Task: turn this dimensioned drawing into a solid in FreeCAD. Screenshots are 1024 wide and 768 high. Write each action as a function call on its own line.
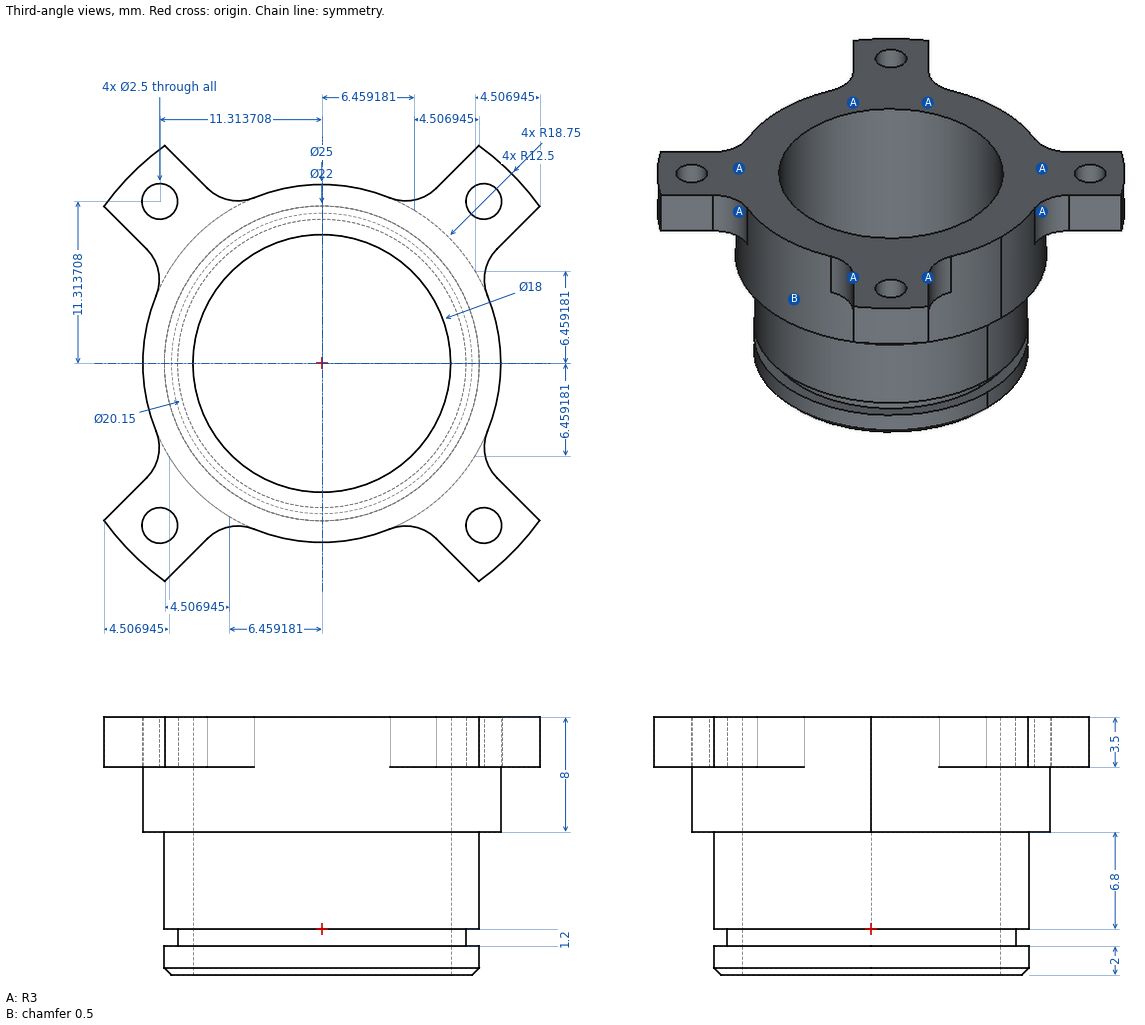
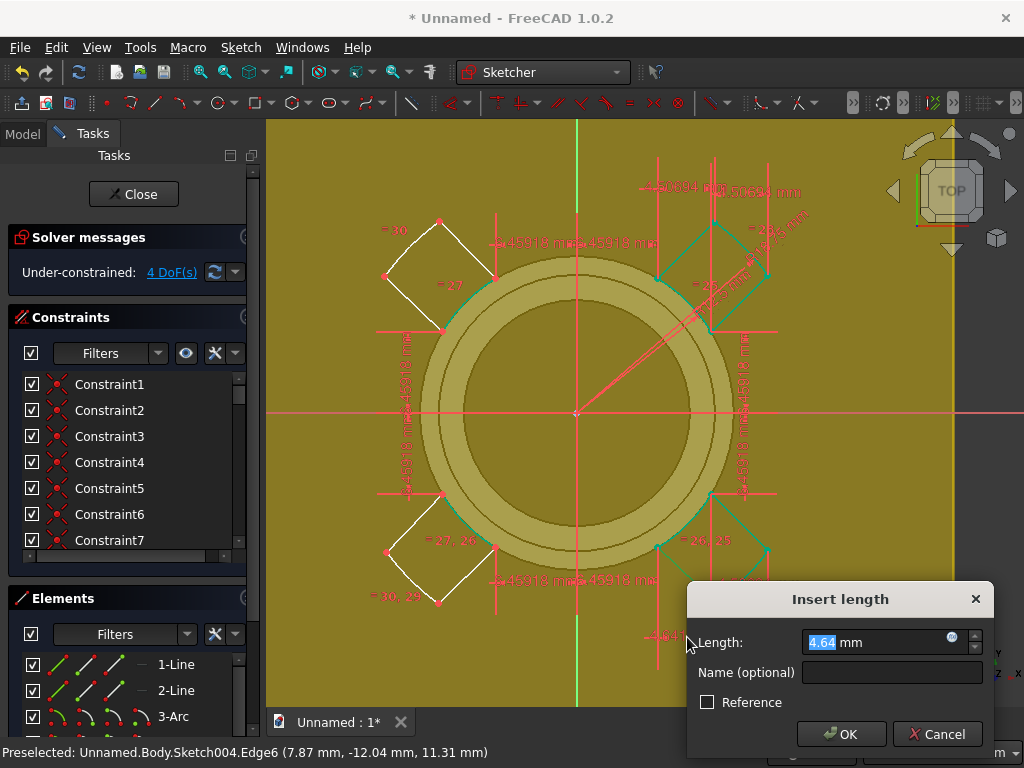
text(4.506945)
key(Return)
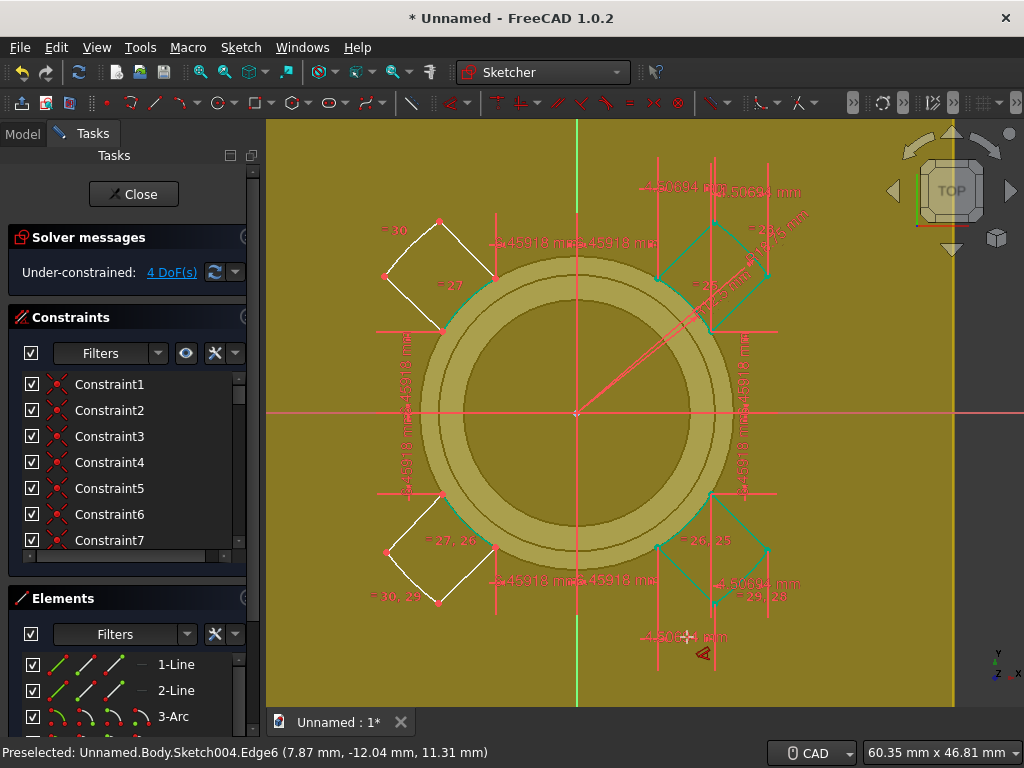
click(456, 587)
click(467, 638)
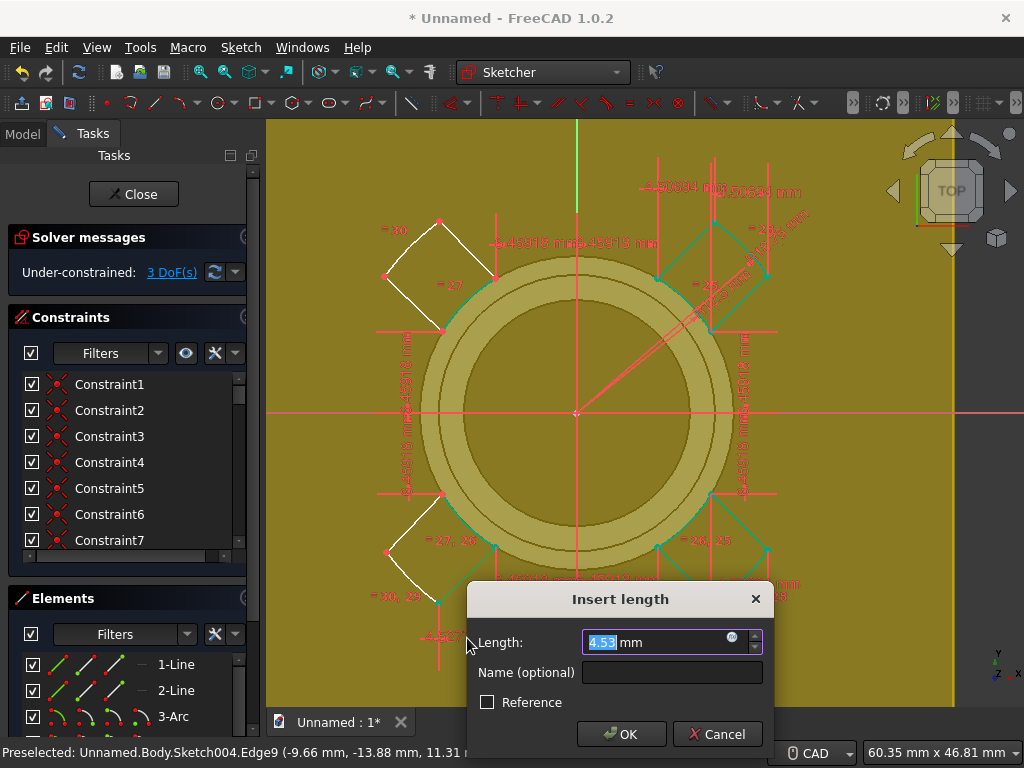
text(4.506945)
key(Return)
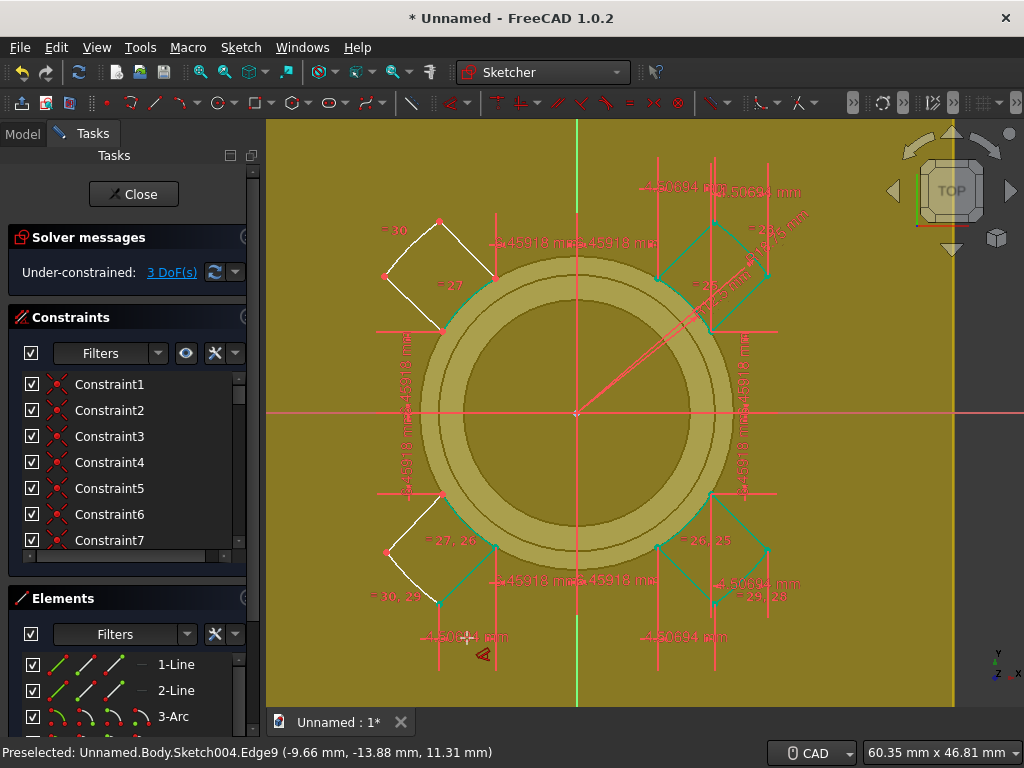
click(426, 512)
click(395, 586)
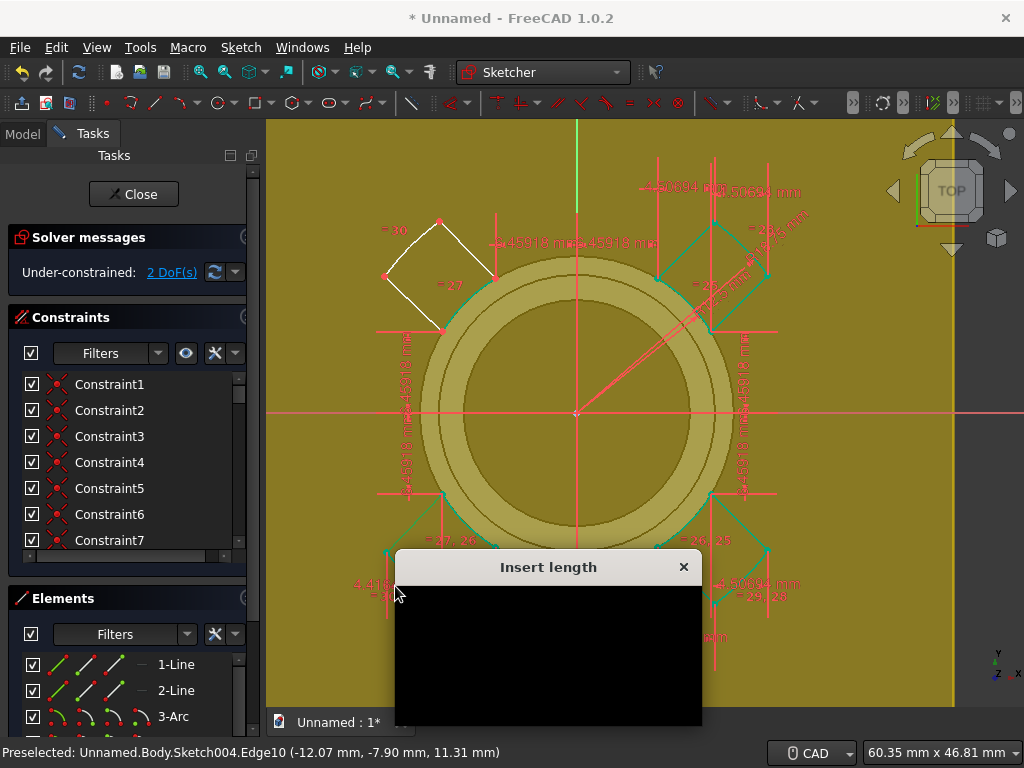
text(4.506945)
key(Return)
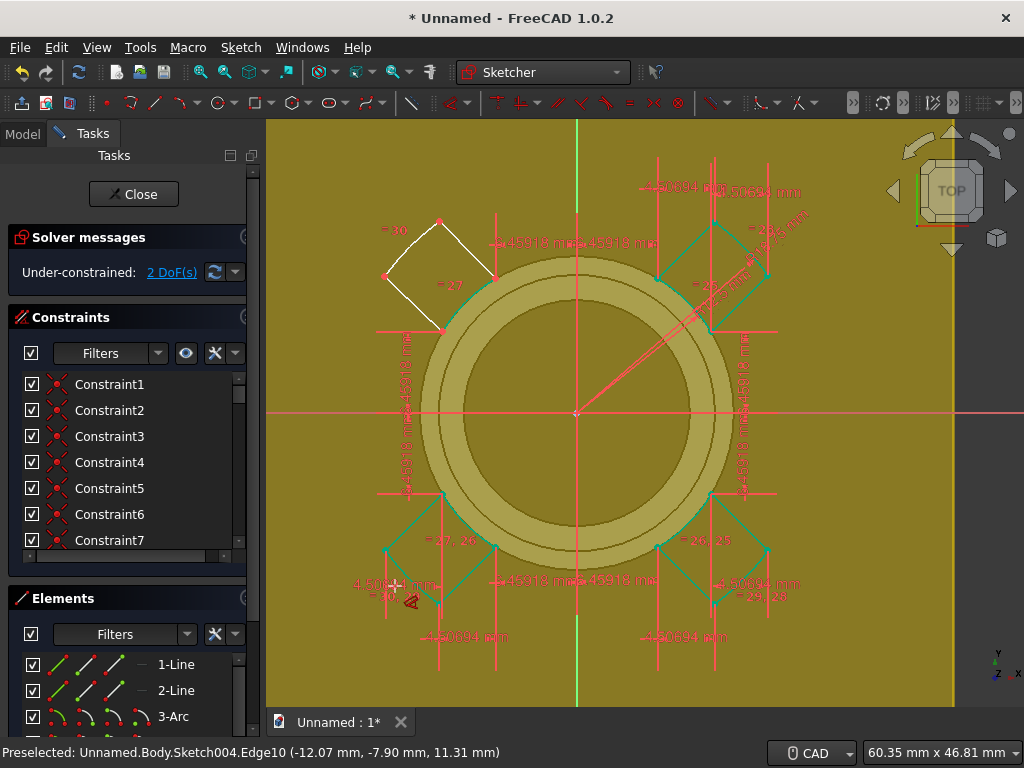
click(402, 293)
click(393, 243)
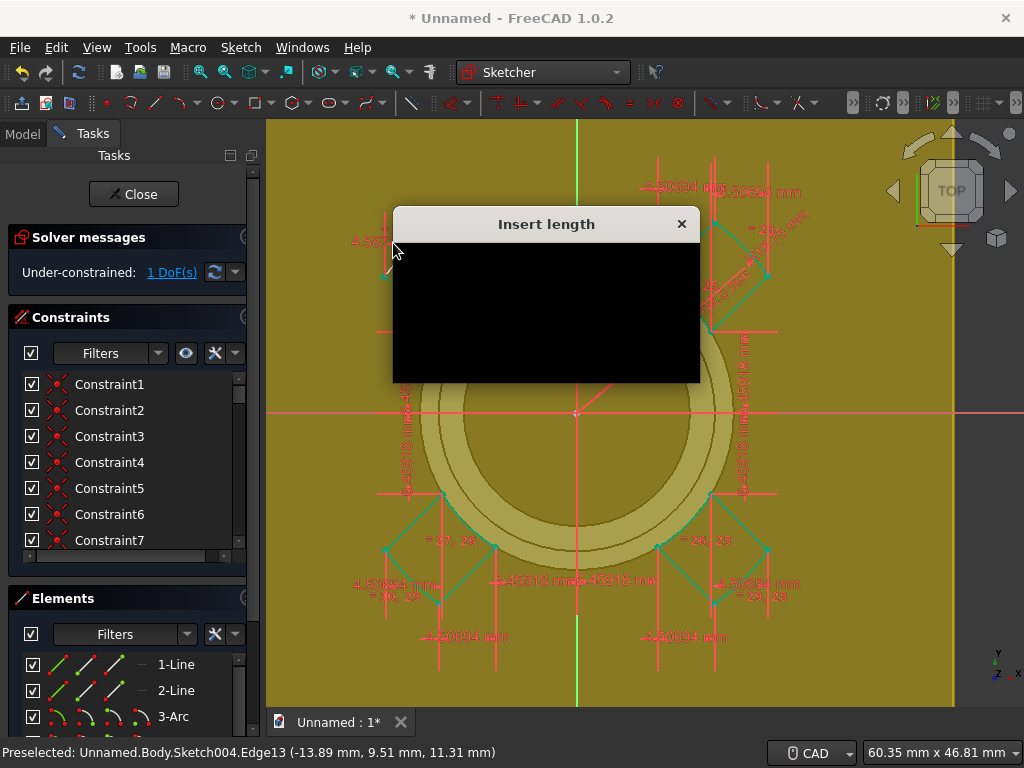
text(4.506945)
key(Return)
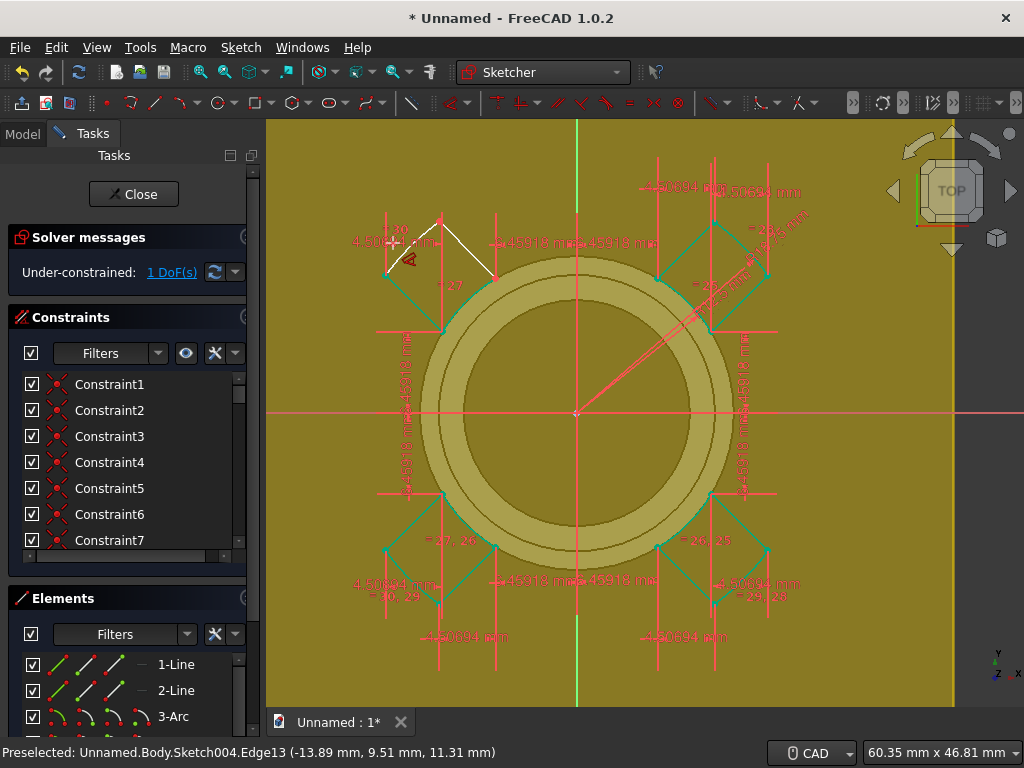
click(479, 262)
click(468, 187)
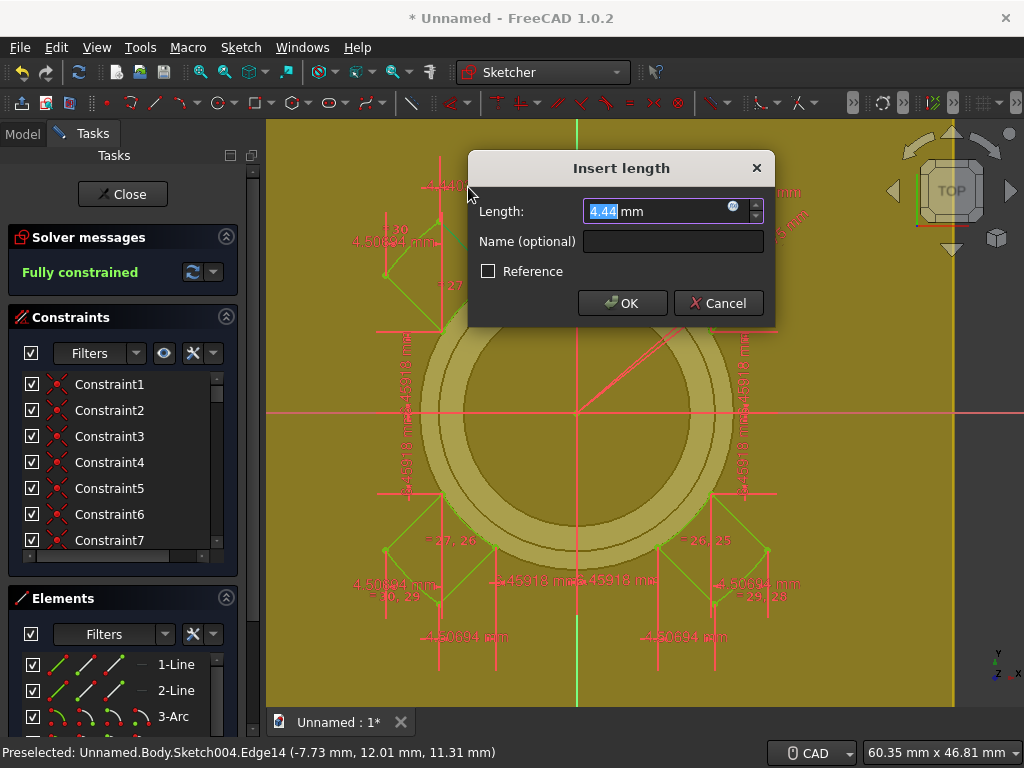
text(4.506945)
key(Return)
key(Escape)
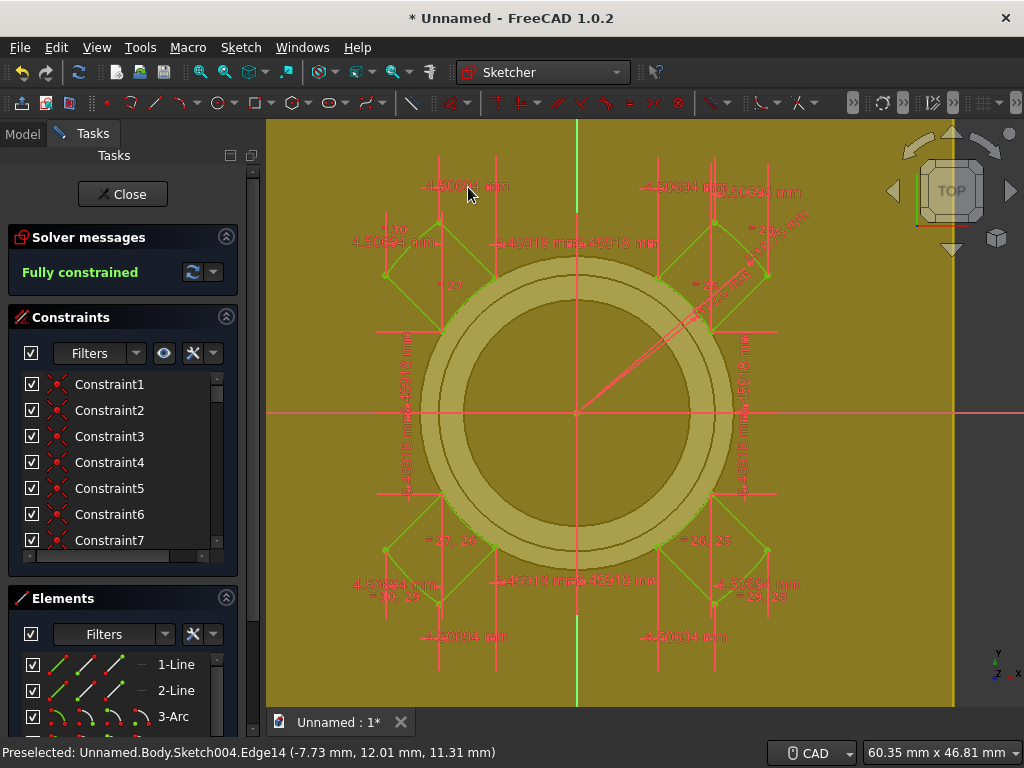
click(123, 194)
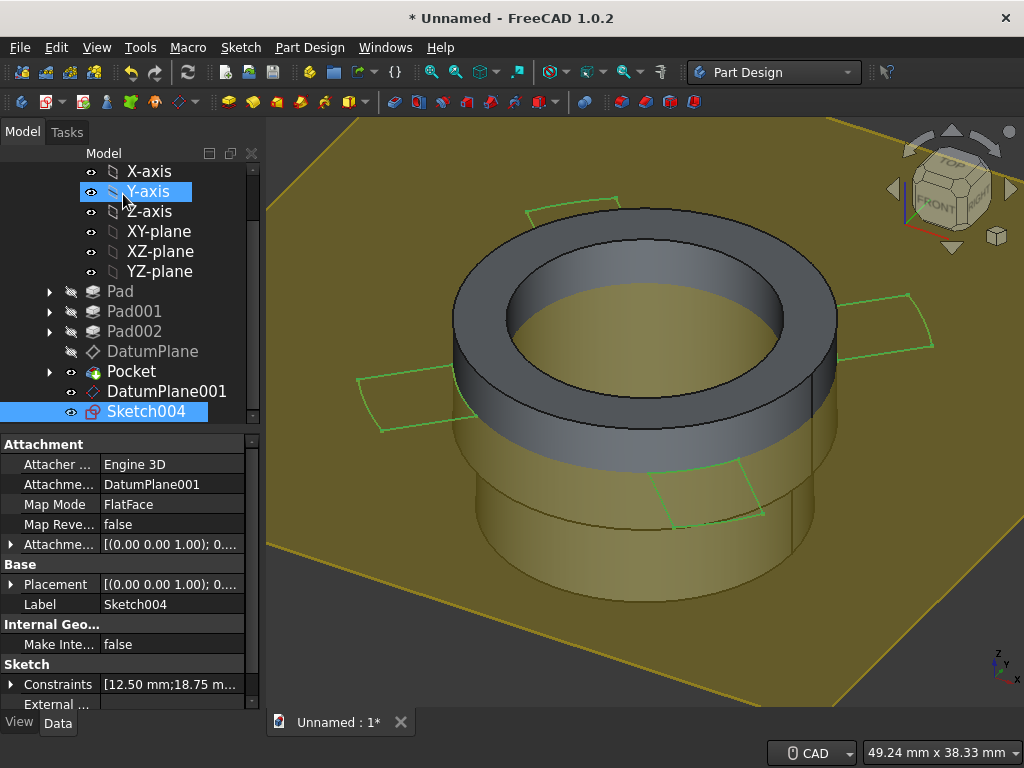
click(230, 102)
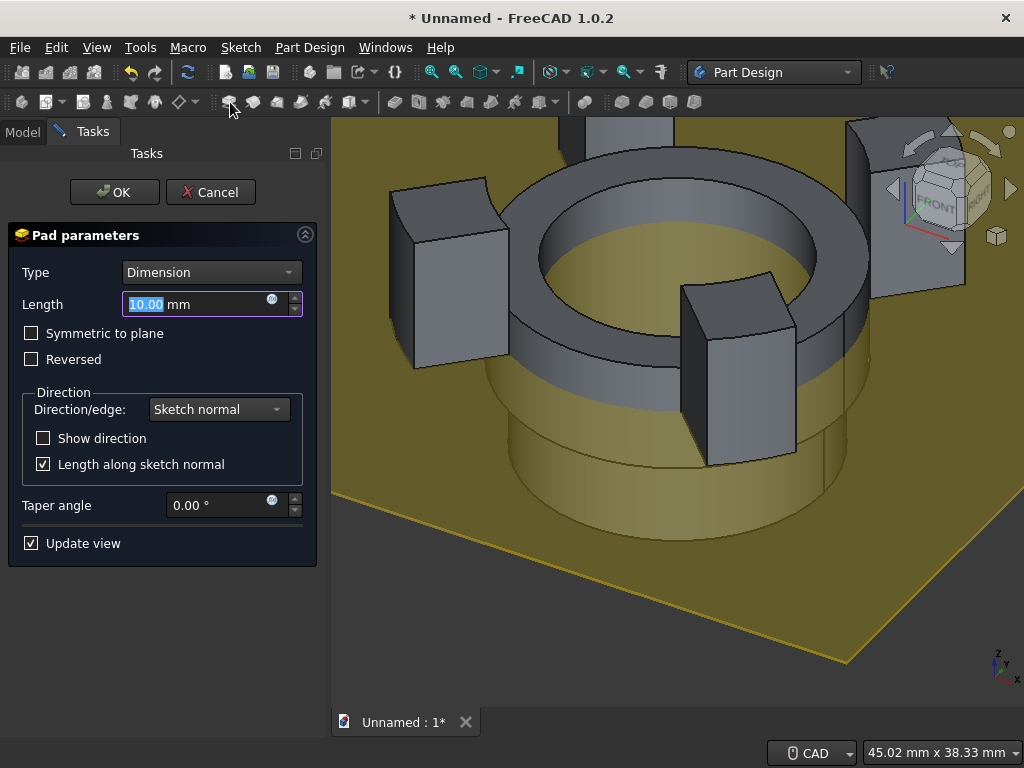
text(3.5)
key(Tab)